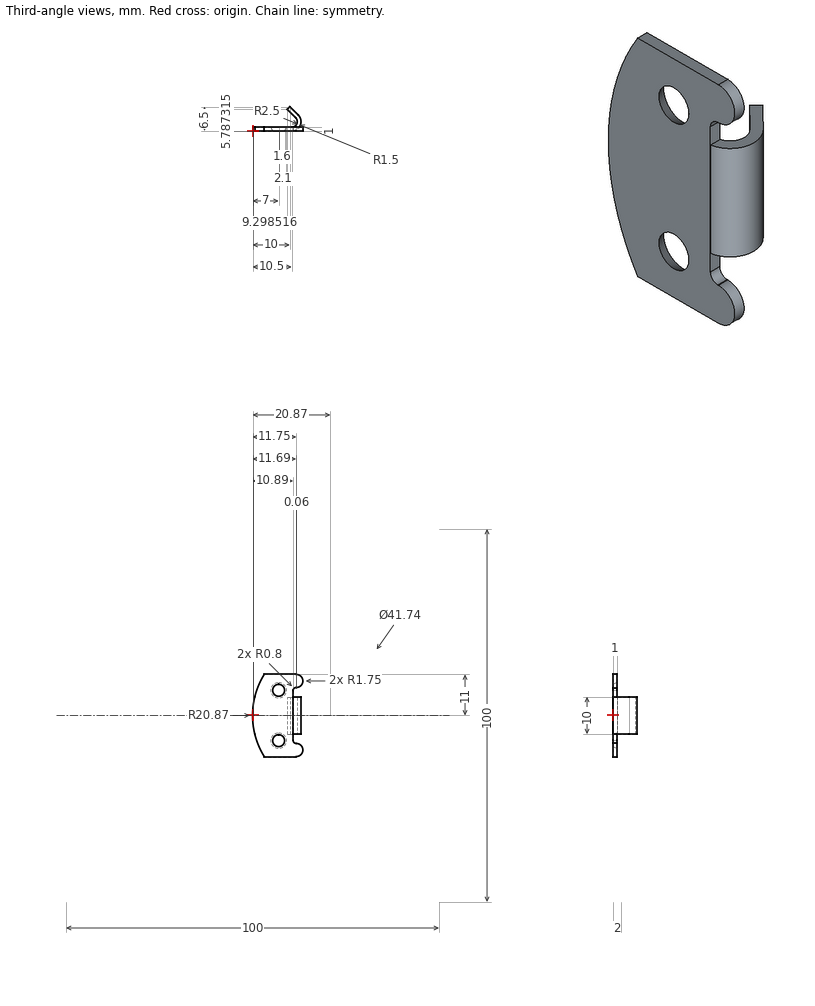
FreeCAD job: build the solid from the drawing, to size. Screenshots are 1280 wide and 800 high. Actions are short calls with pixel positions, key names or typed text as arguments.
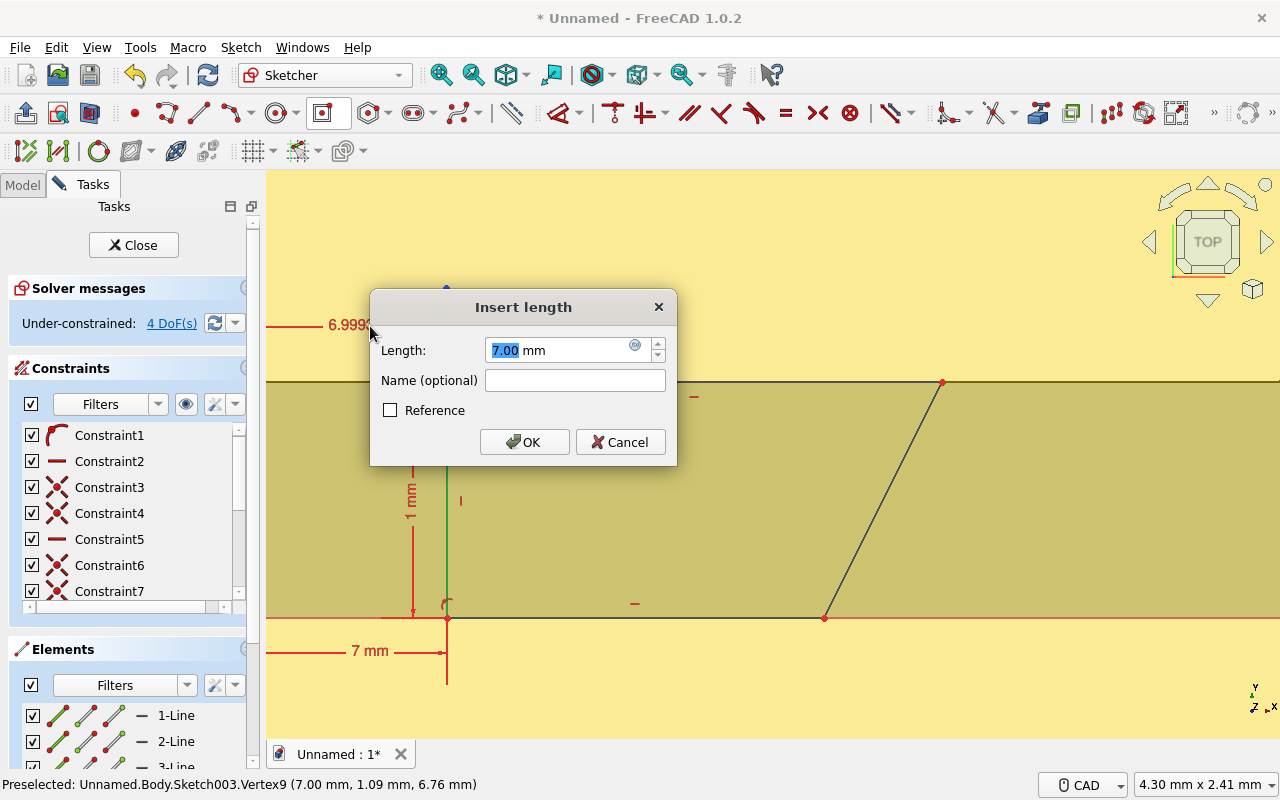
text(7)
key(Return)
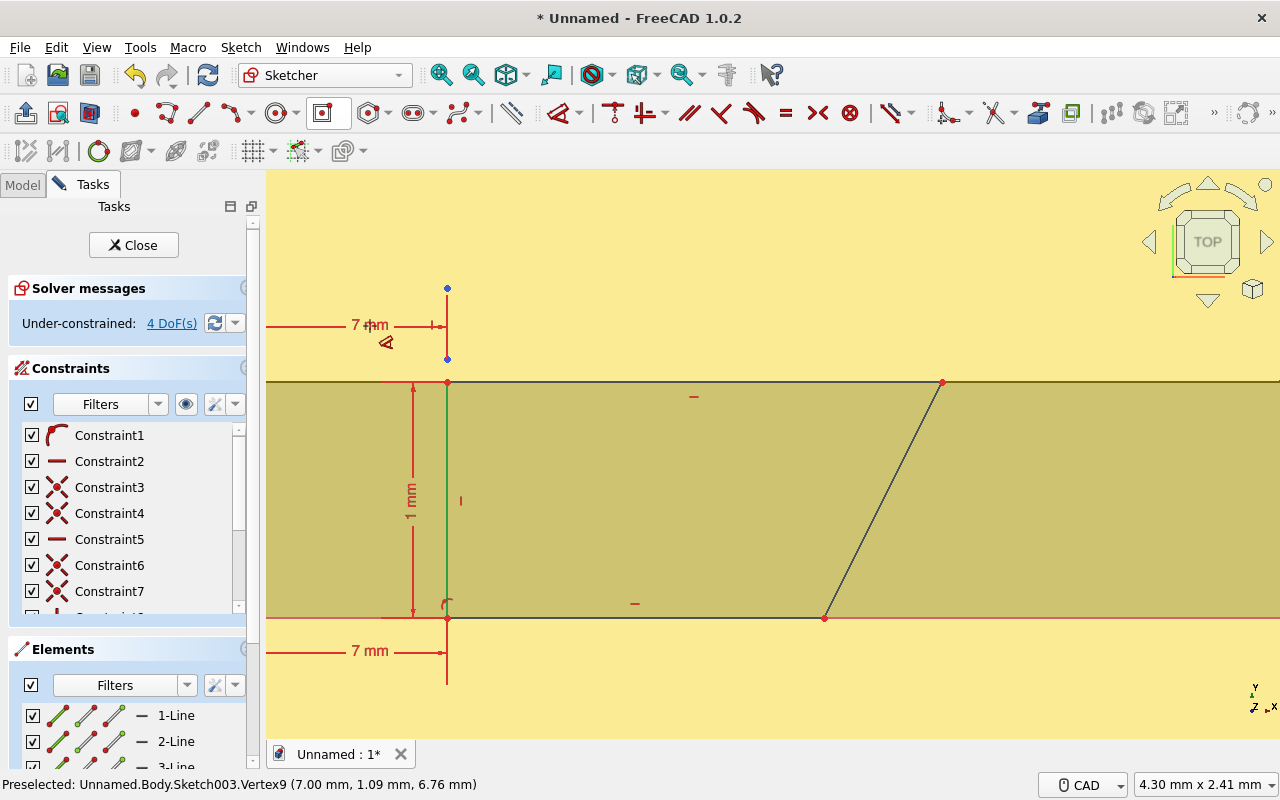
click(560, 618)
click(636, 652)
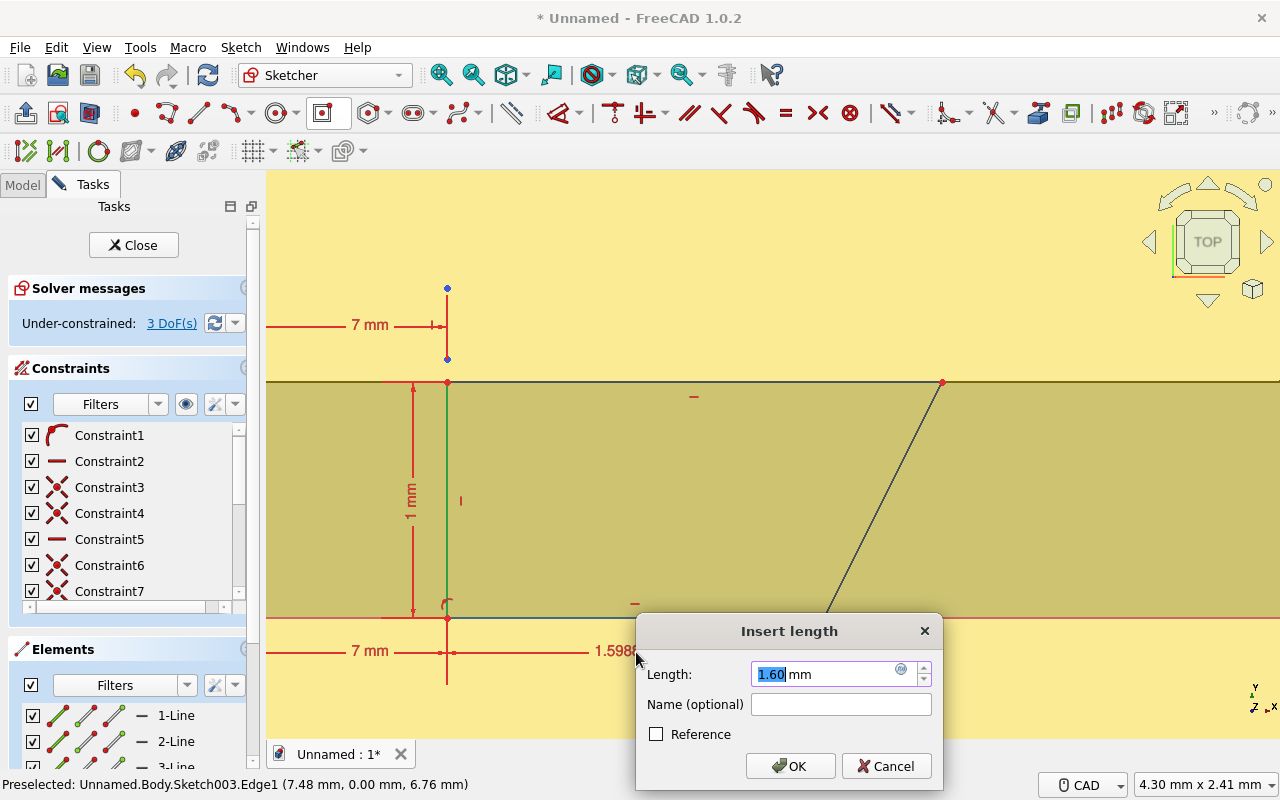
text(1.6)
key(Return)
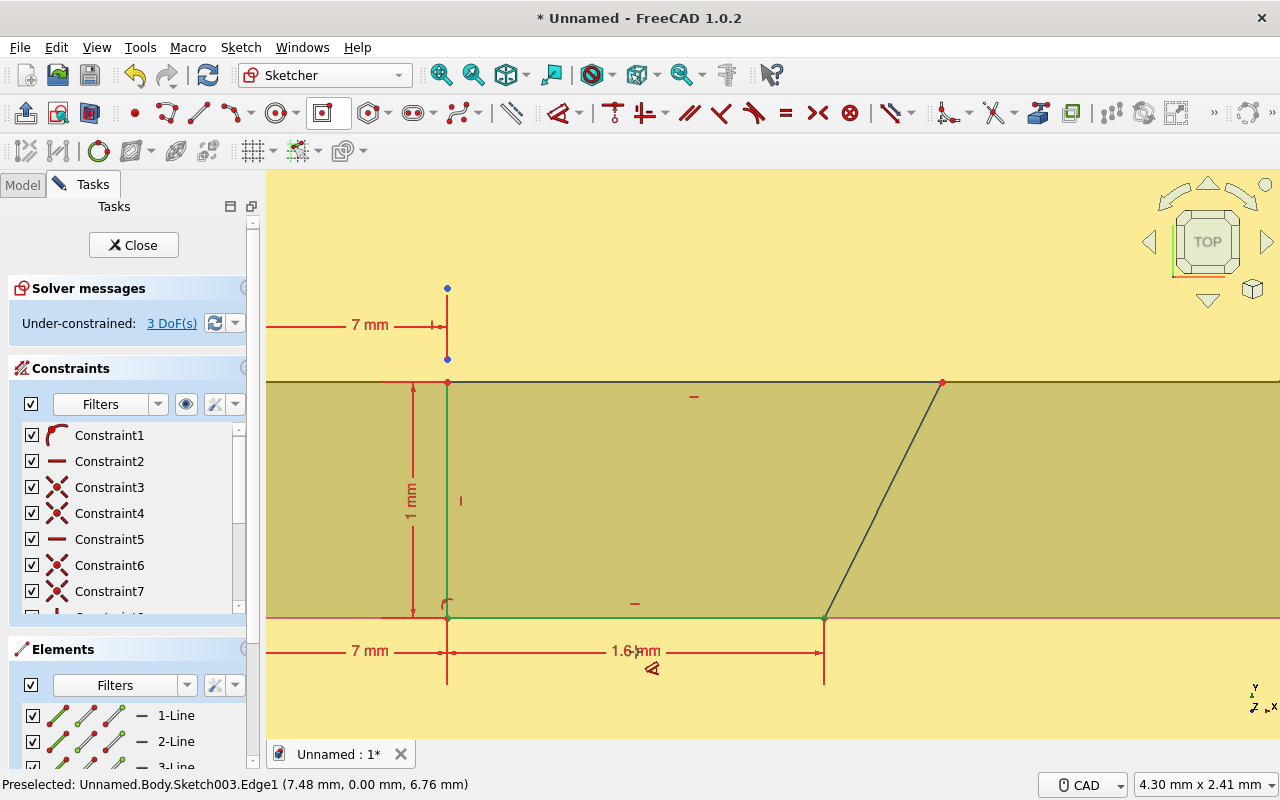
click(794, 382)
click(695, 348)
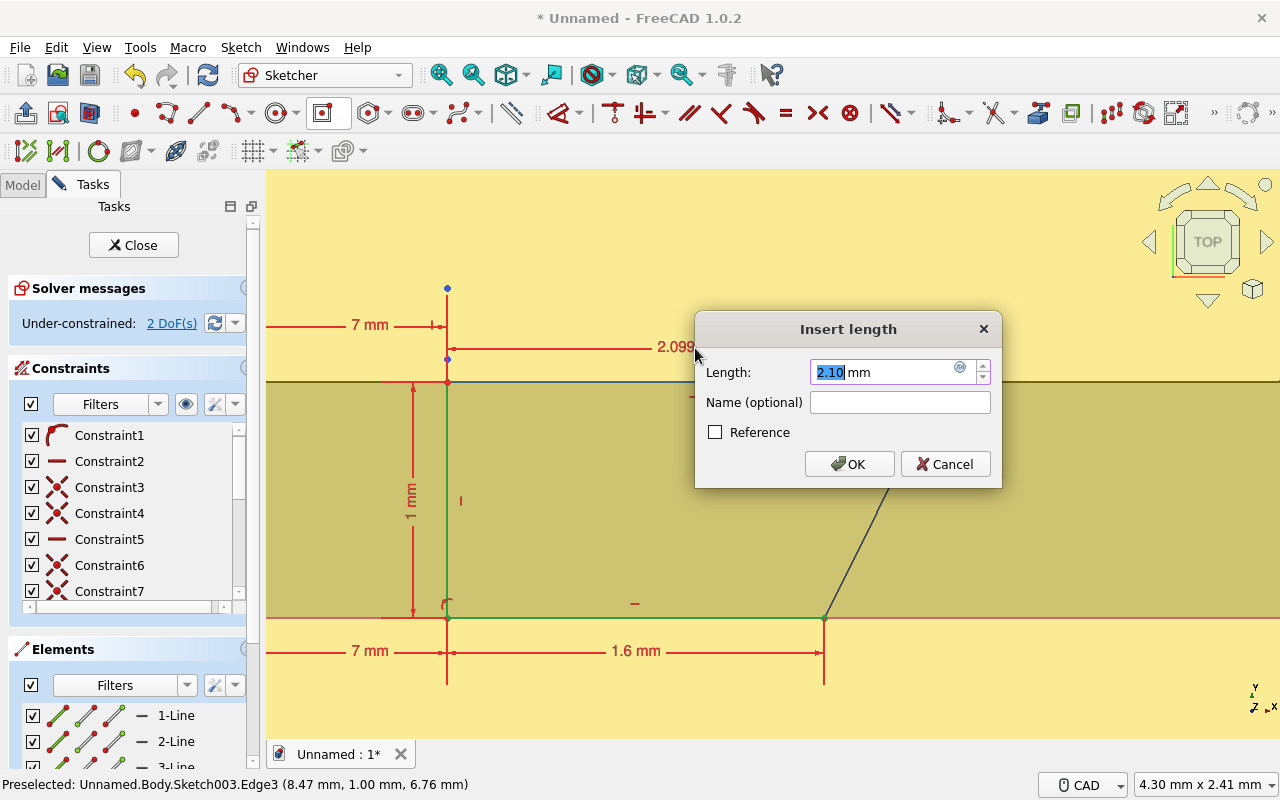
text(2.1)
key(Return)
key(Escape)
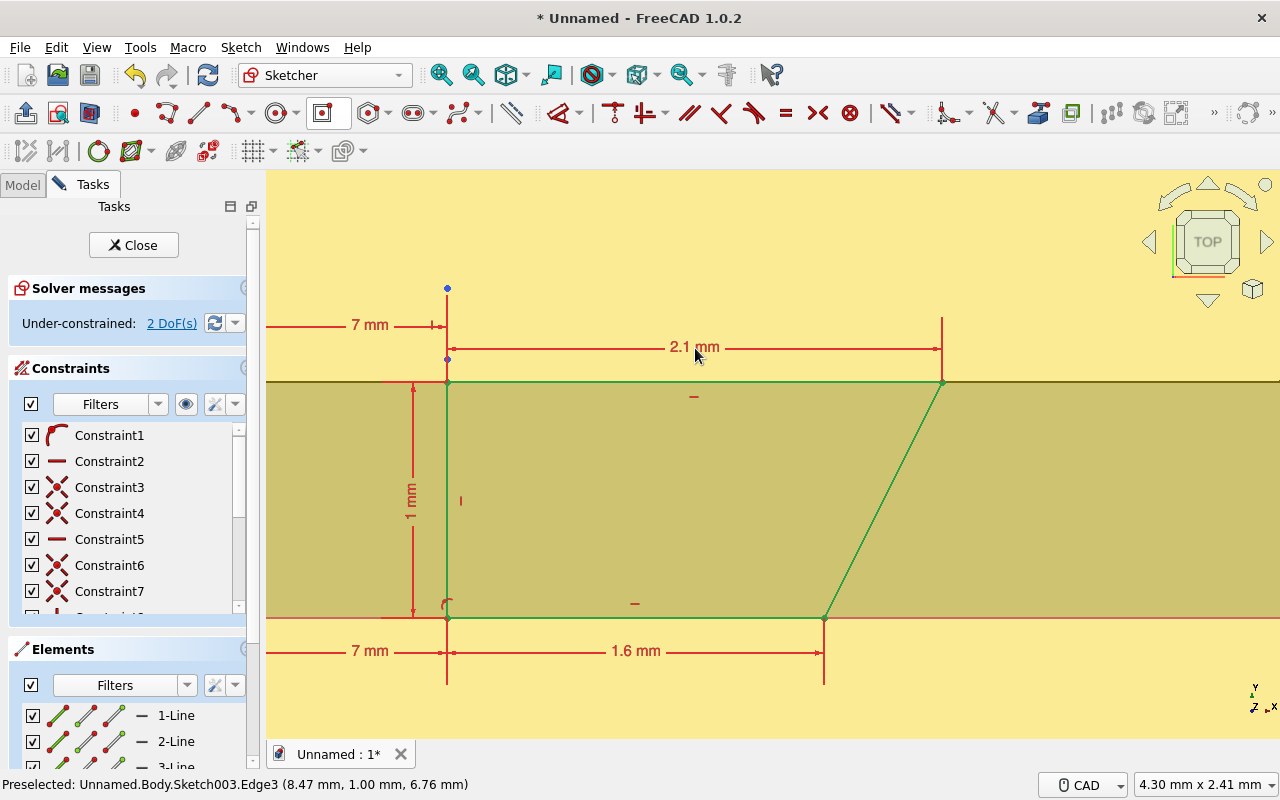
click(134, 245)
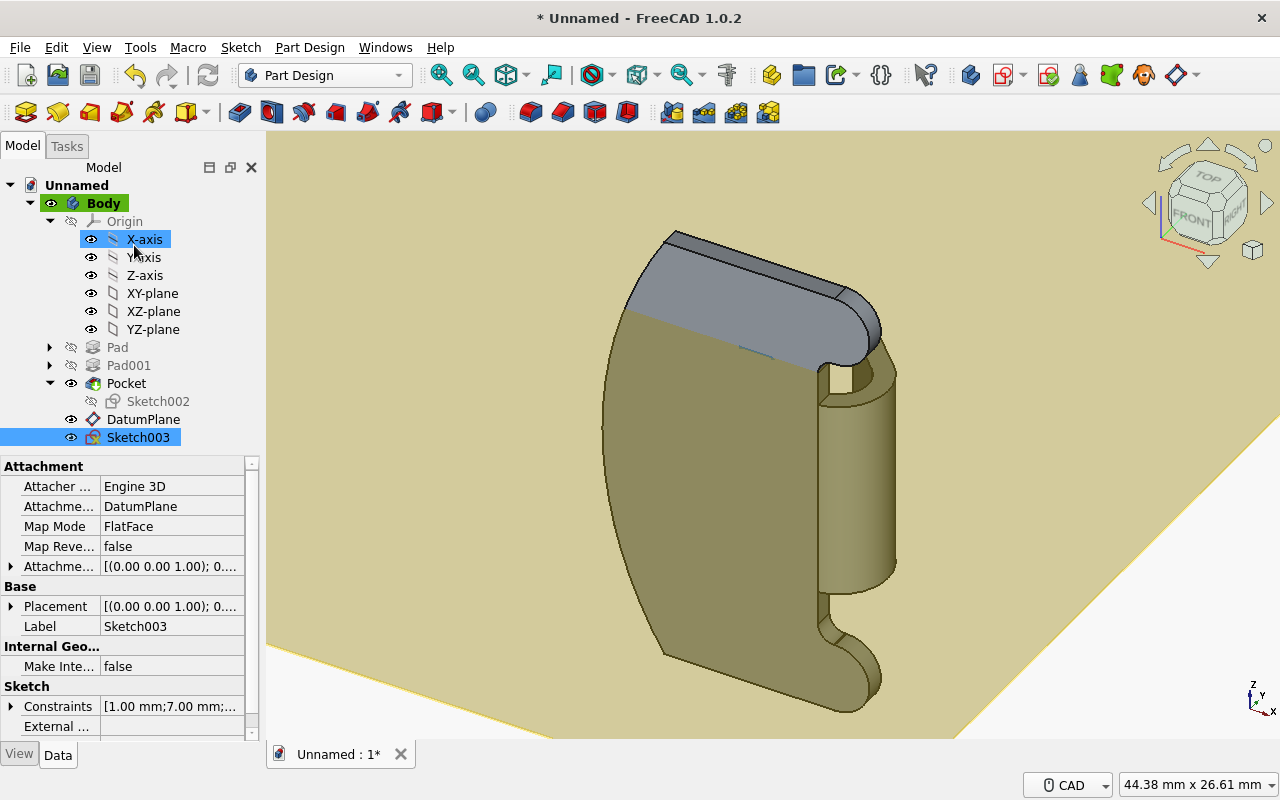
click(304, 112)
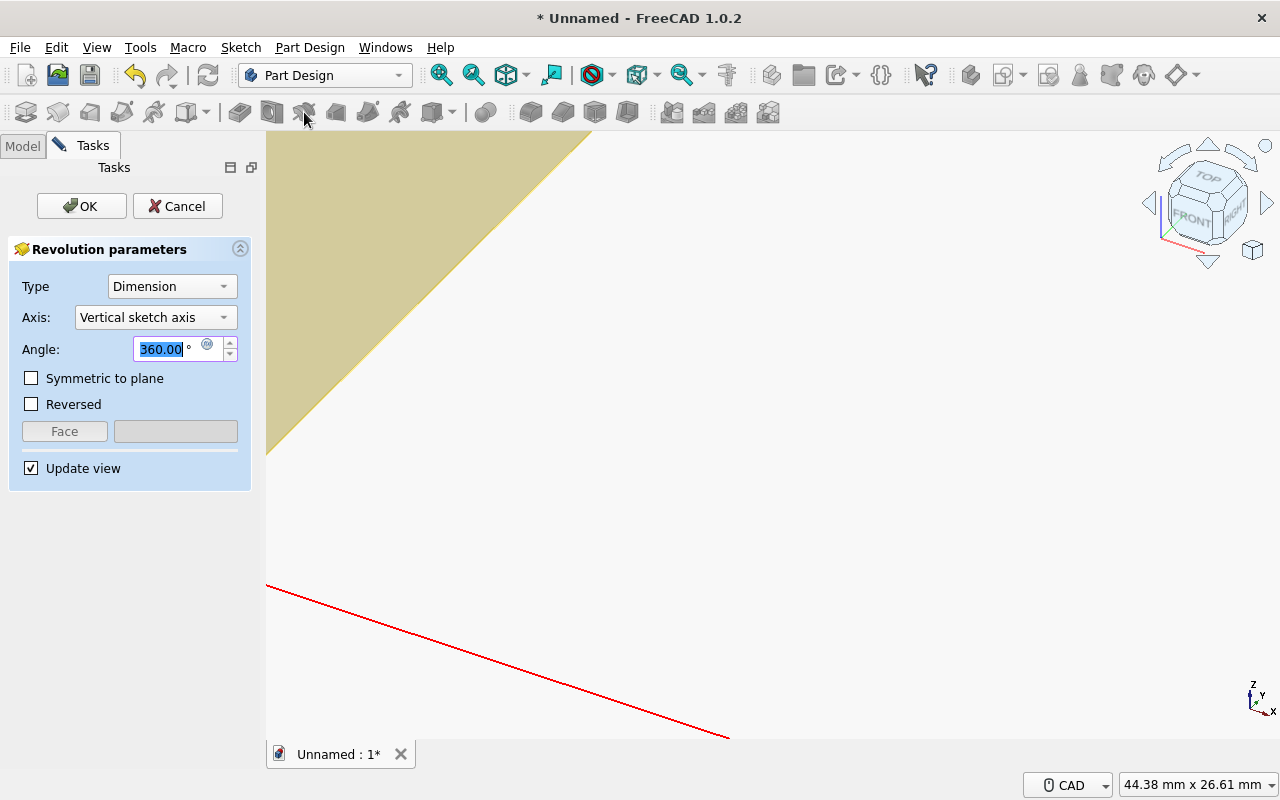
click(156, 318)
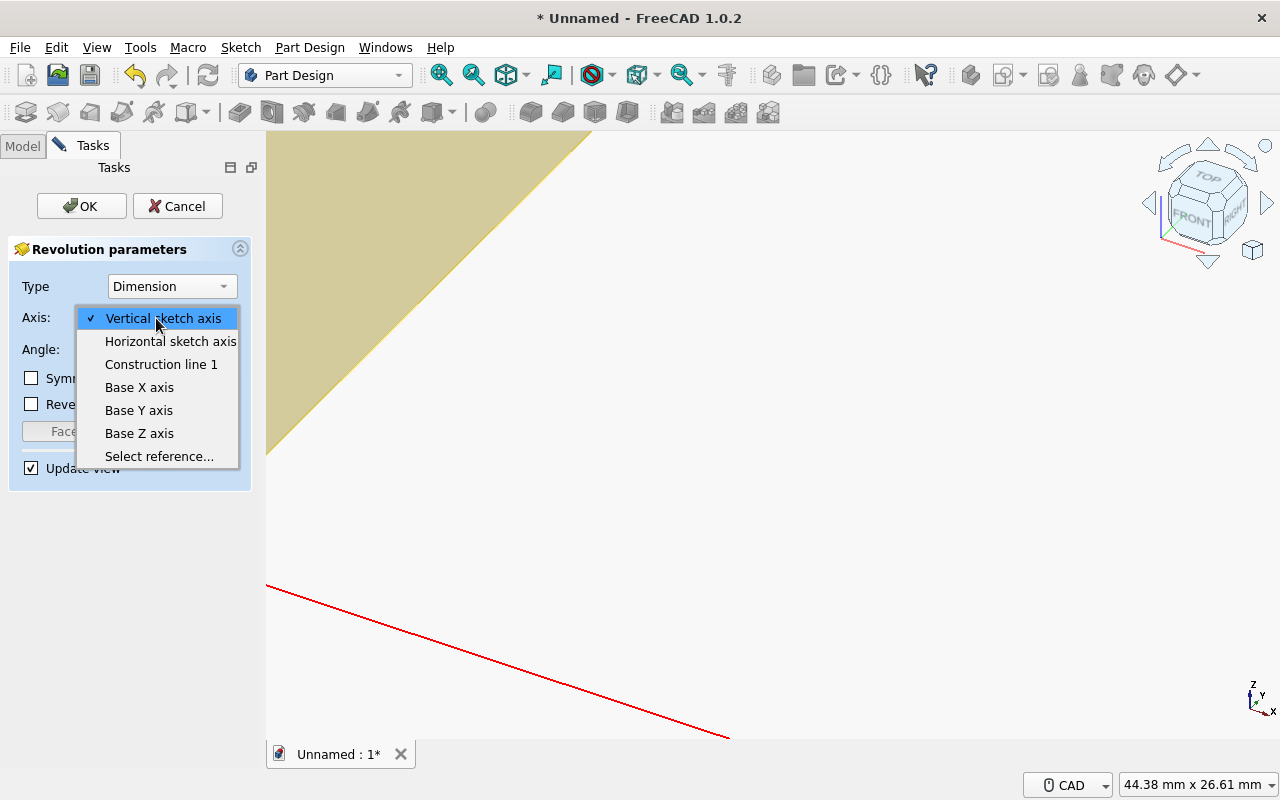
click(156, 364)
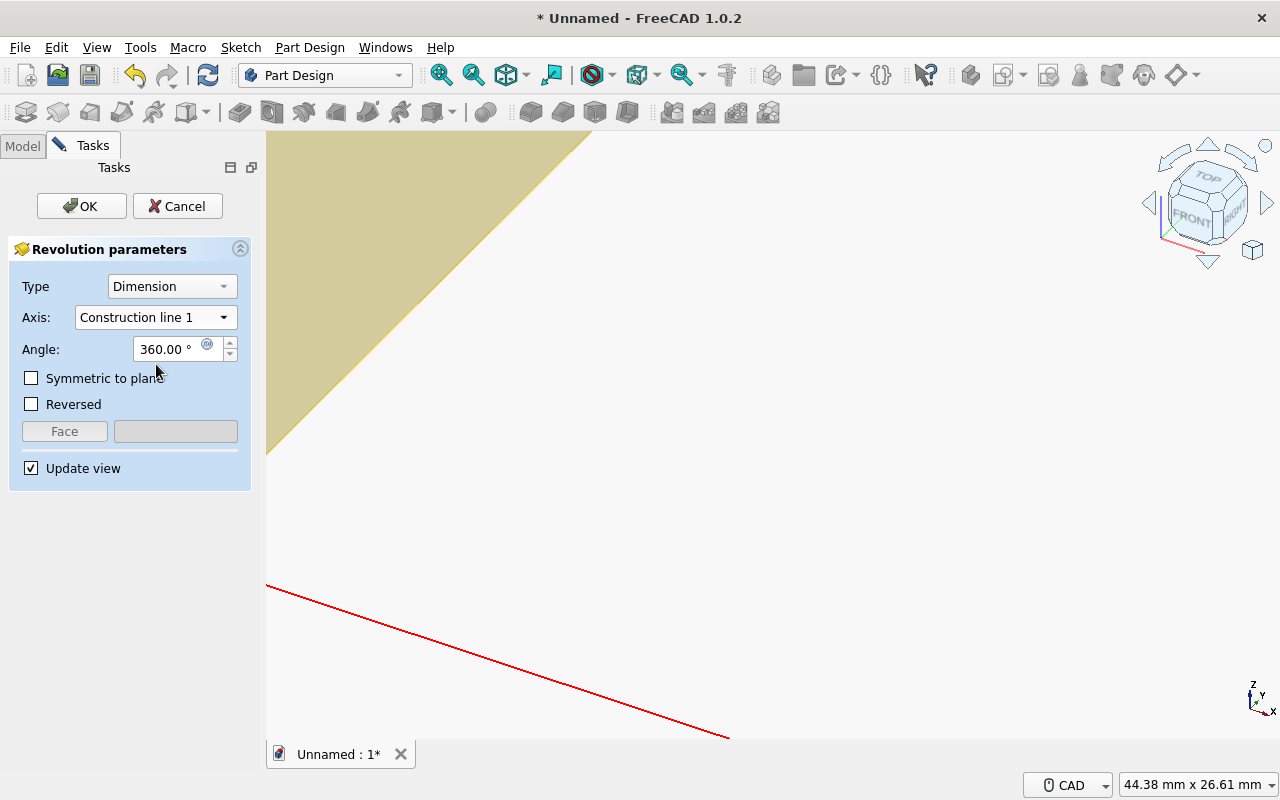
click(82, 206)